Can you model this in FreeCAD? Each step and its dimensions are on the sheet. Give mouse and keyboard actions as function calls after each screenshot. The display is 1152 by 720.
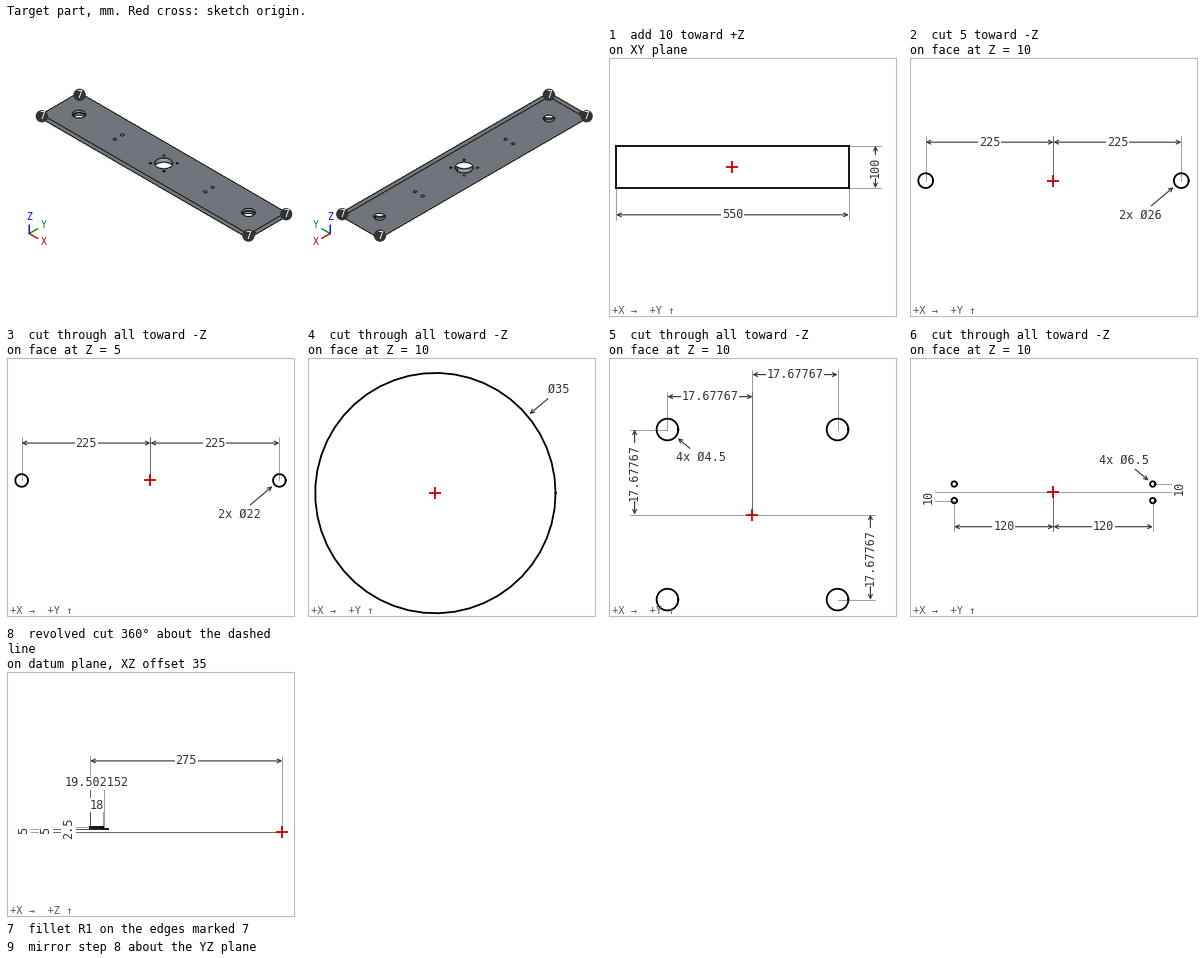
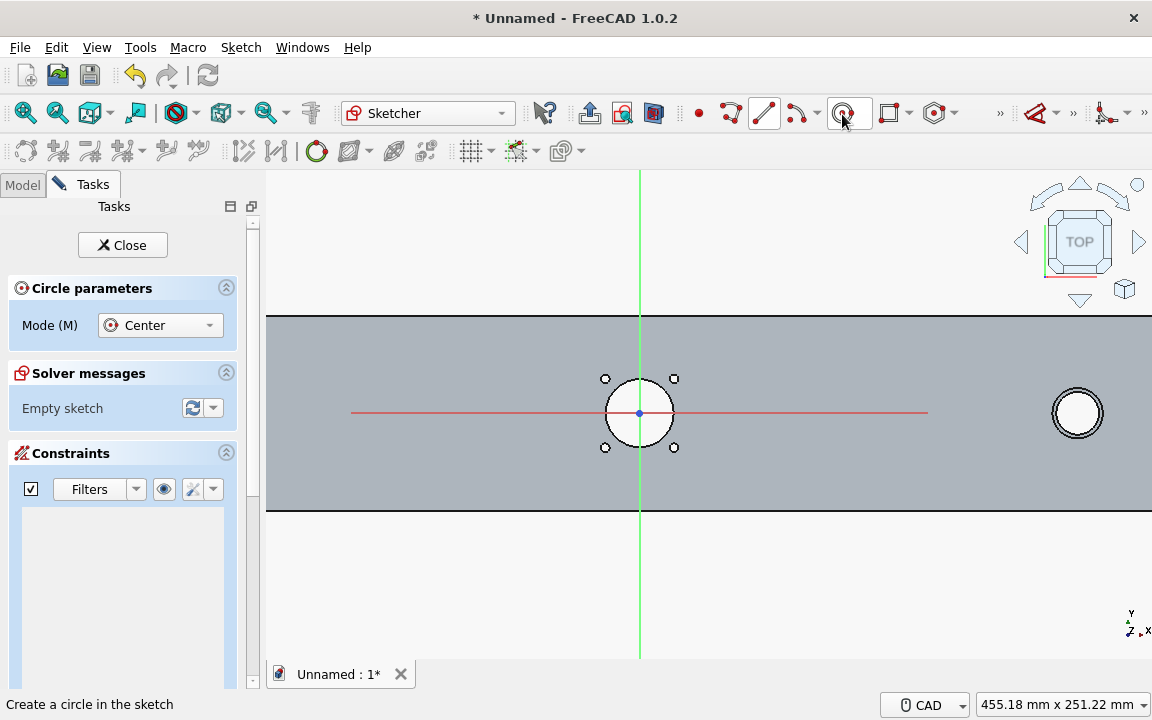
scroll(406, 433, up, 7)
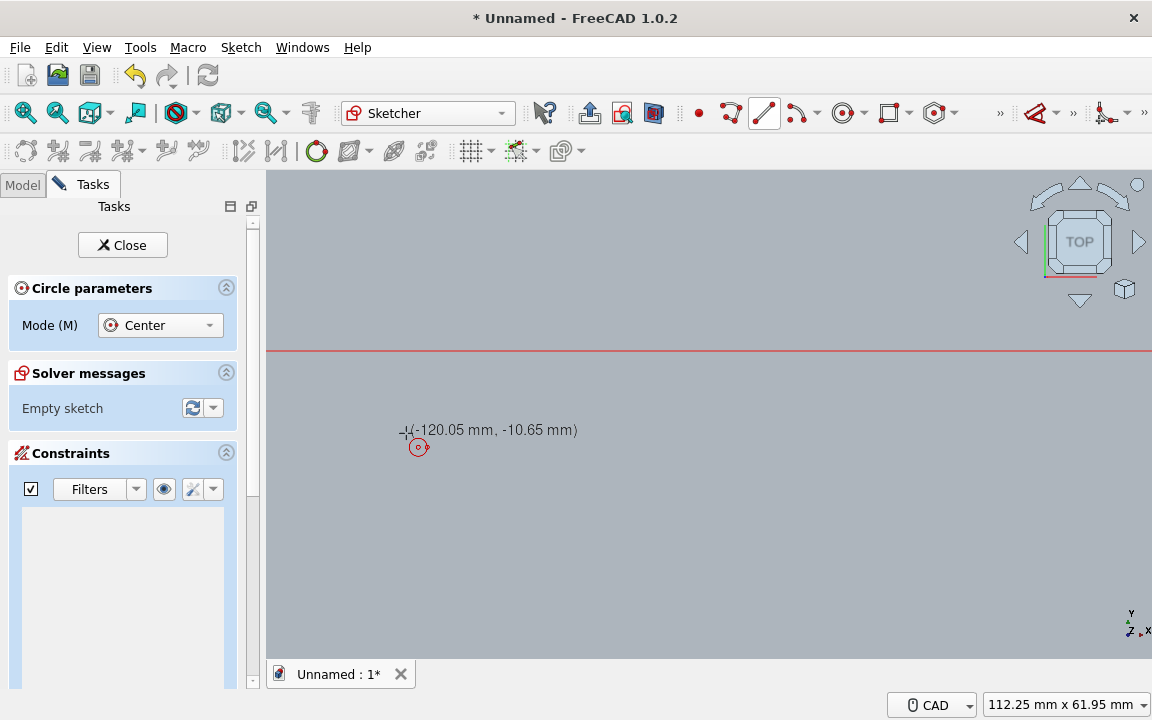
scroll(407, 435, down, 7)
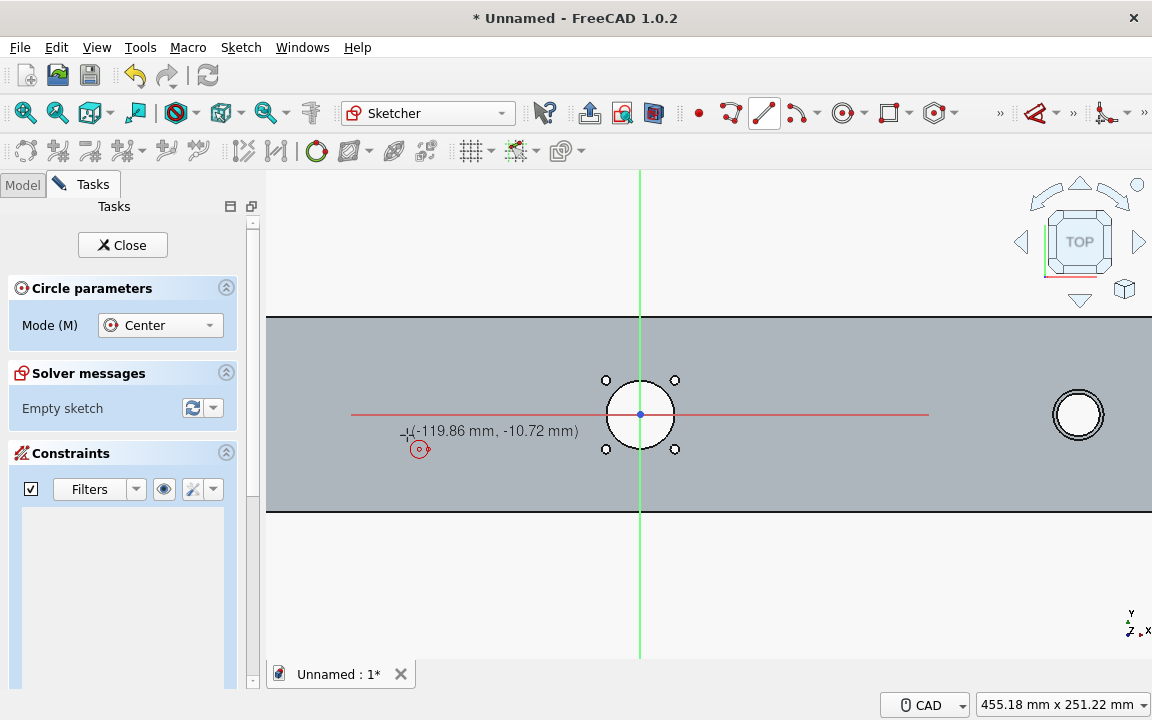
click(407, 434)
move(411, 430)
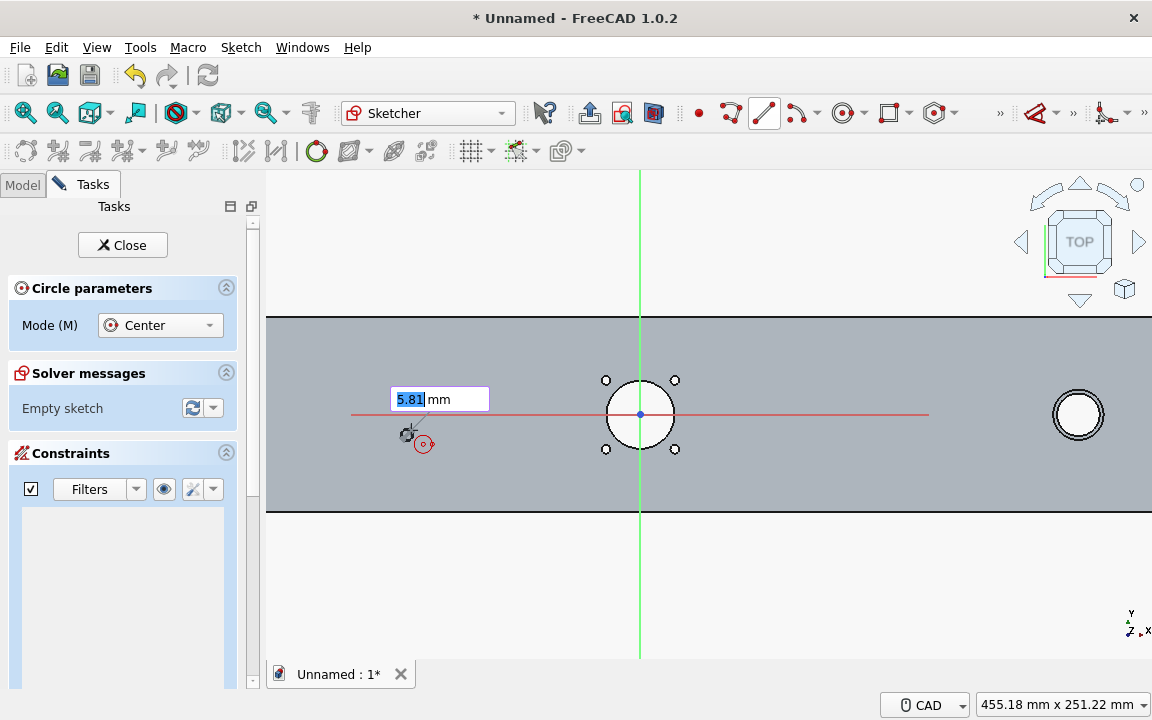
text(6.5)
key(Return)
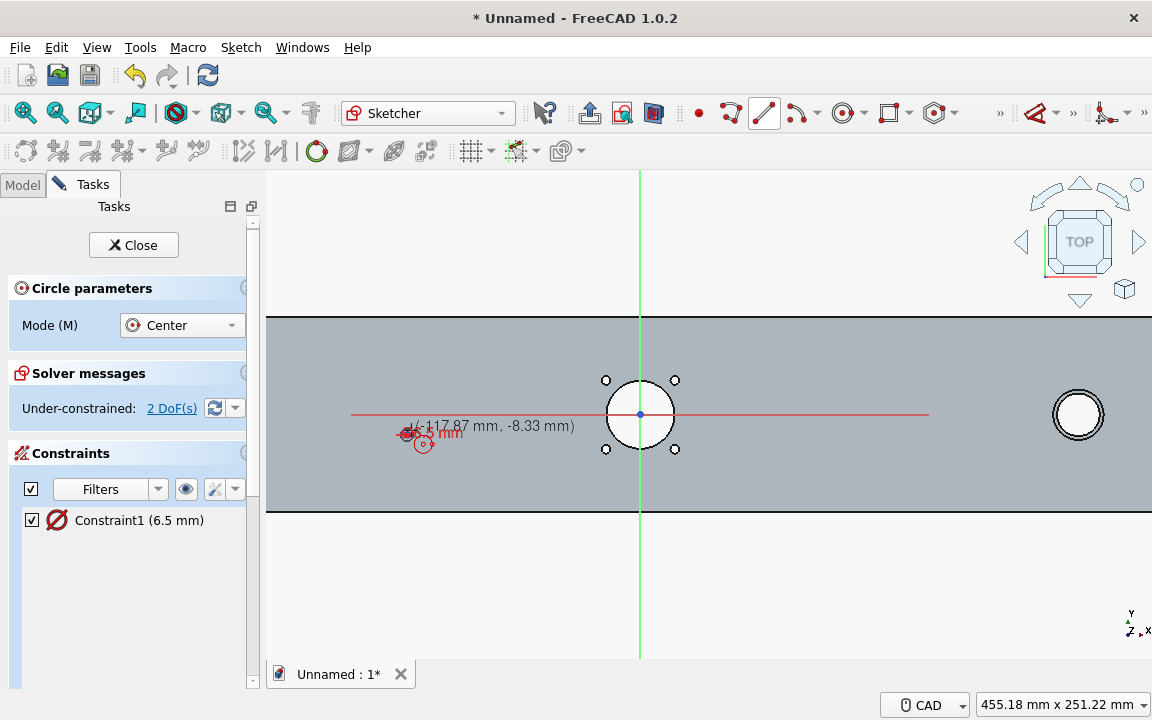
scroll(874, 434, up, 7)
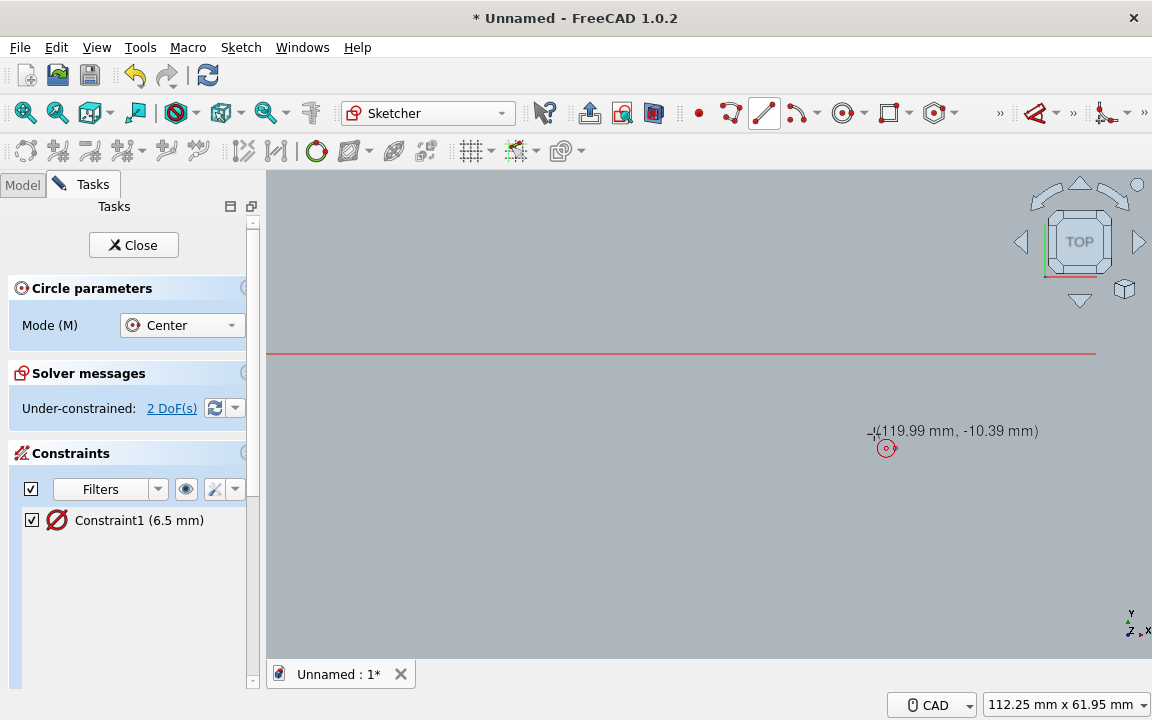
scroll(875, 434, down, 7)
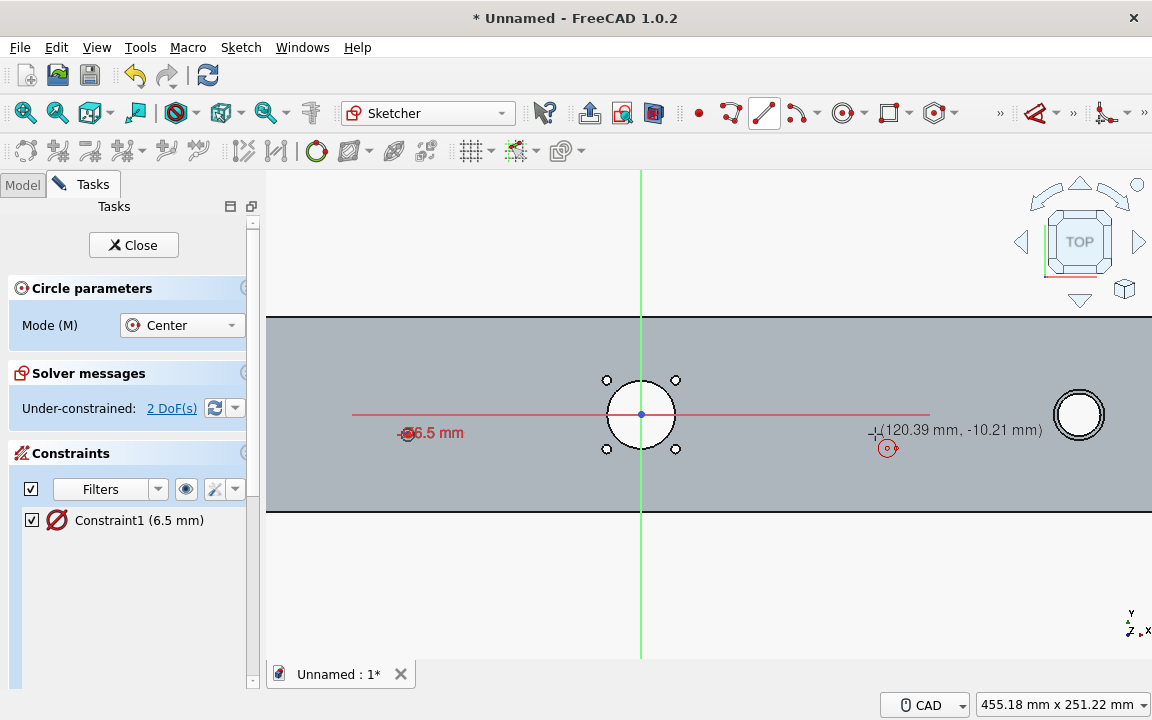
click(875, 434)
move(879, 430)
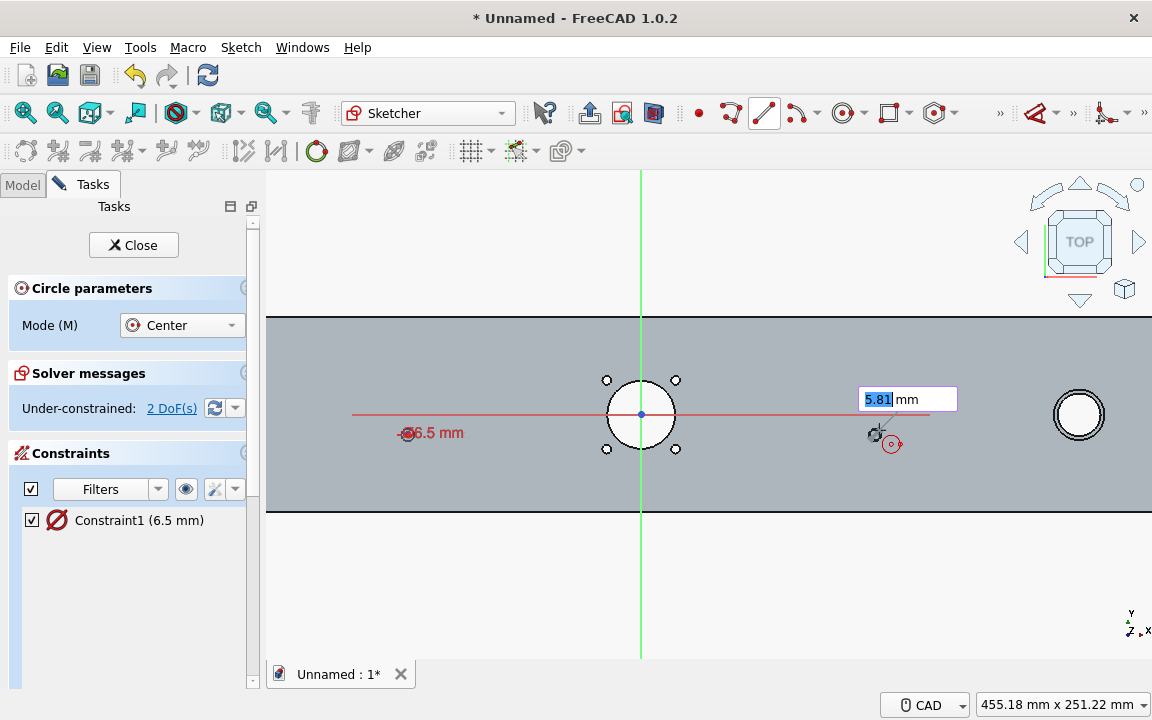
text(6.5)
key(Return)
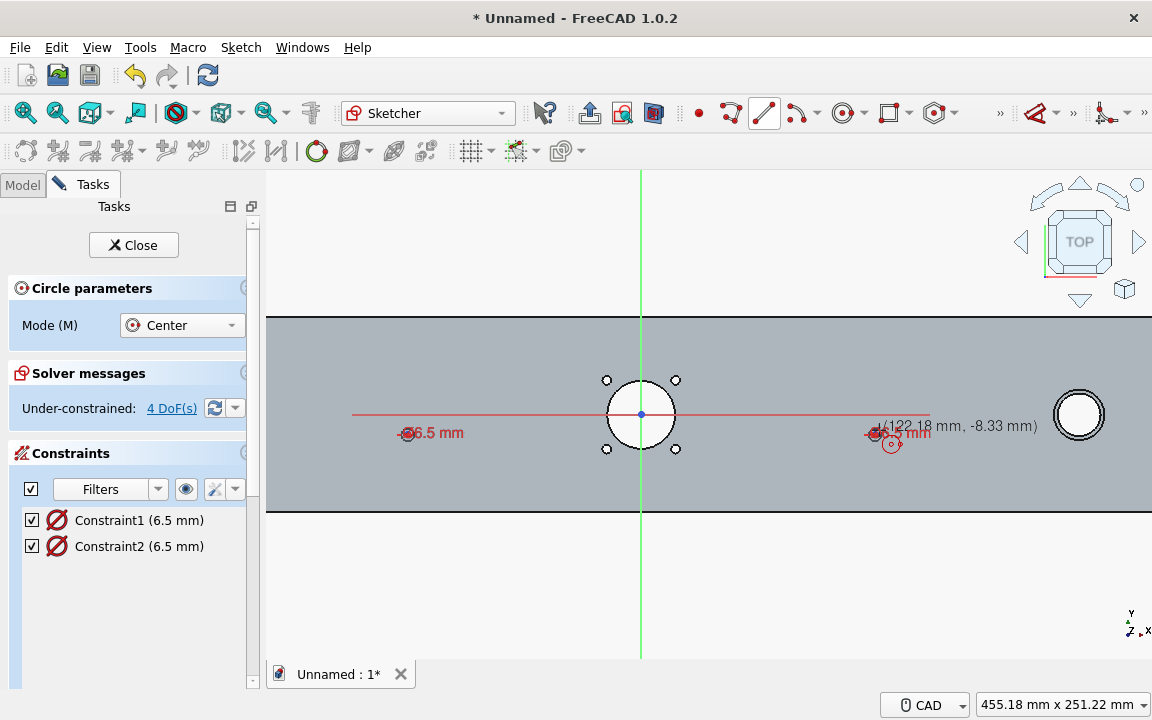
scroll(875, 395, up, 7)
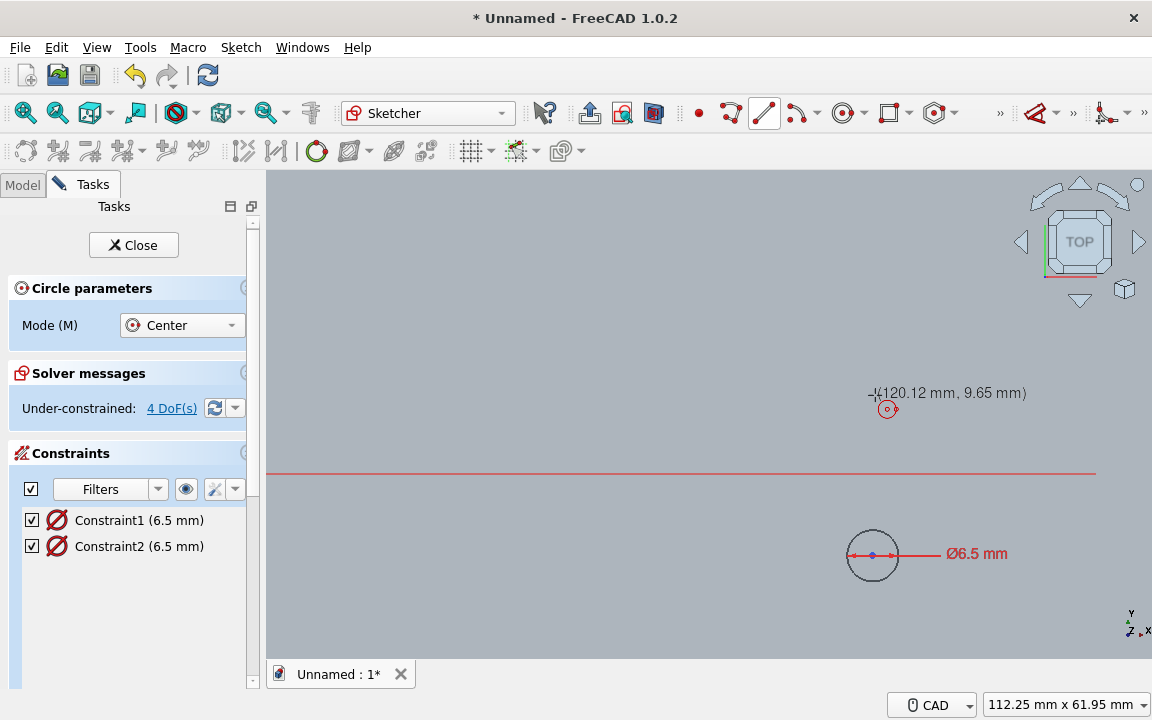
scroll(875, 395, down, 7)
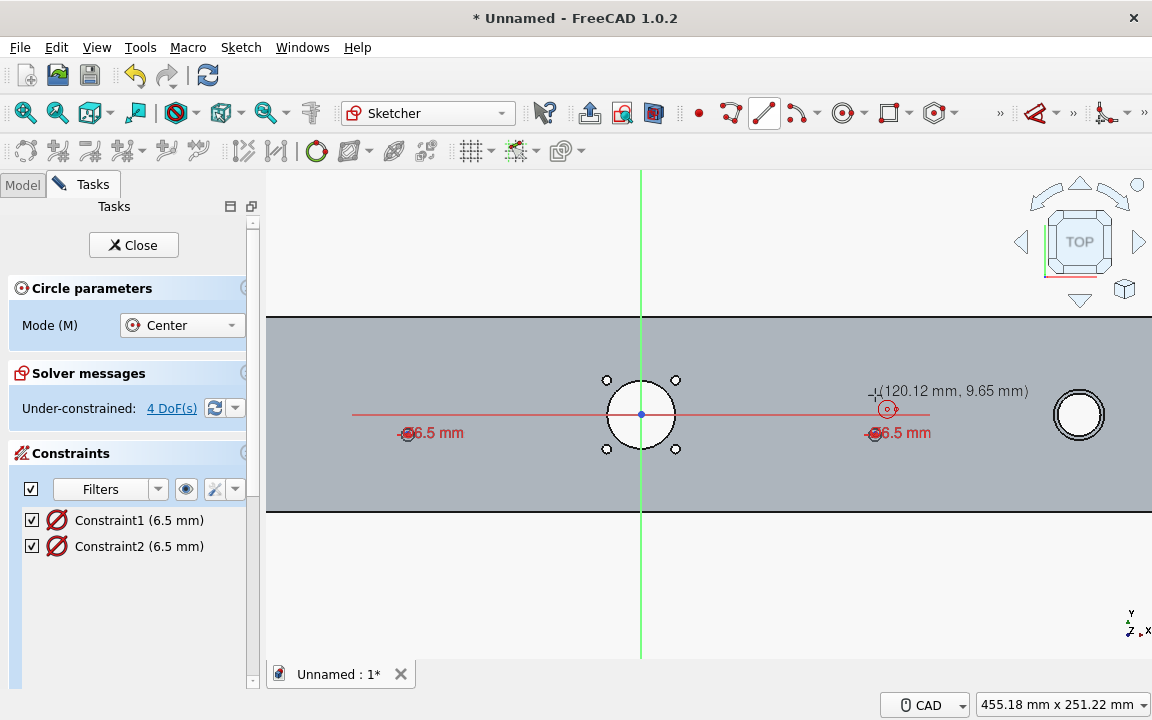
click(875, 395)
move(879, 391)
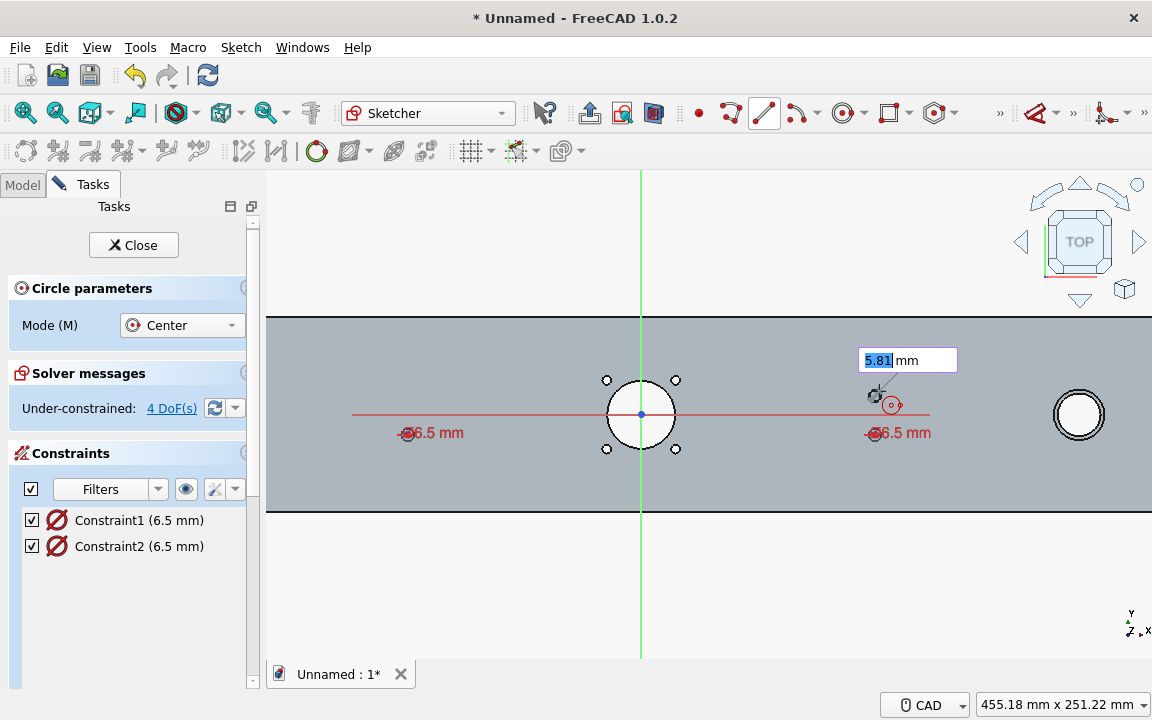
text(6.5)
key(Return)